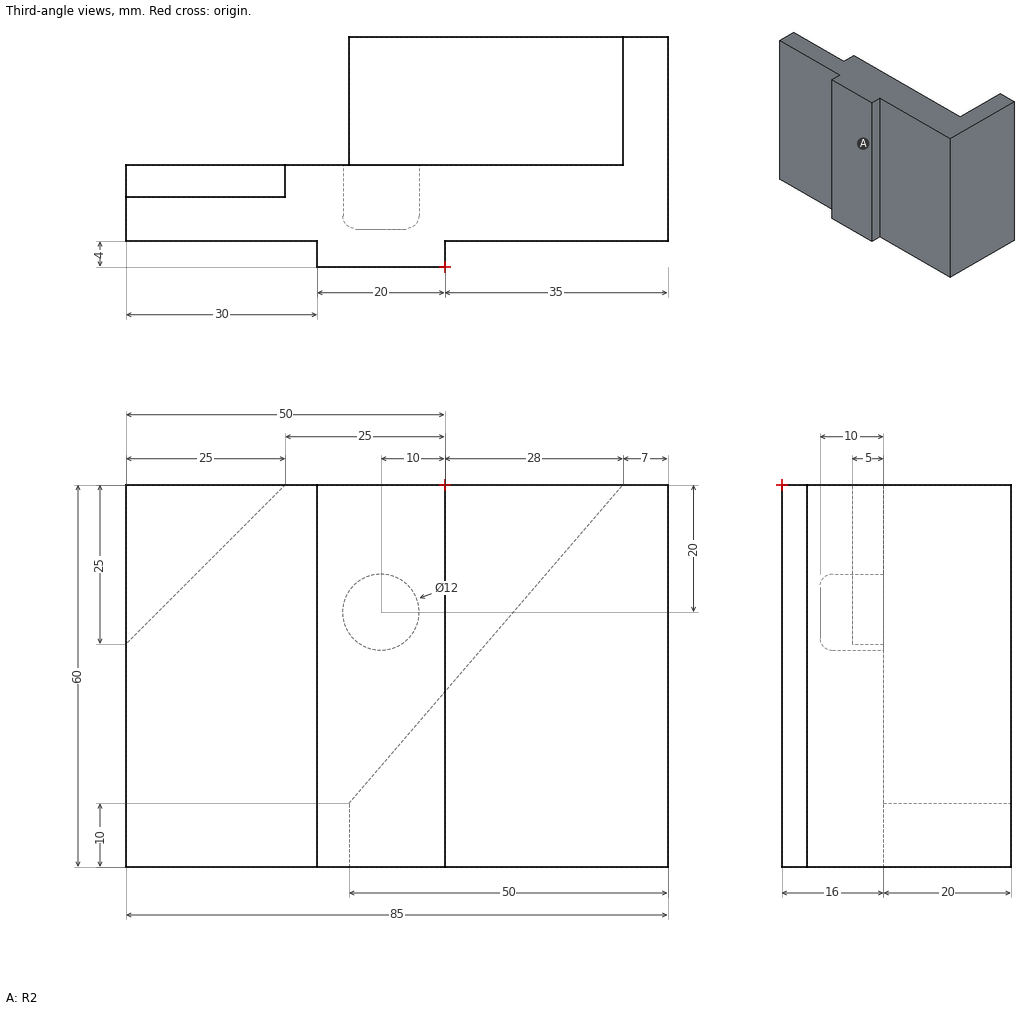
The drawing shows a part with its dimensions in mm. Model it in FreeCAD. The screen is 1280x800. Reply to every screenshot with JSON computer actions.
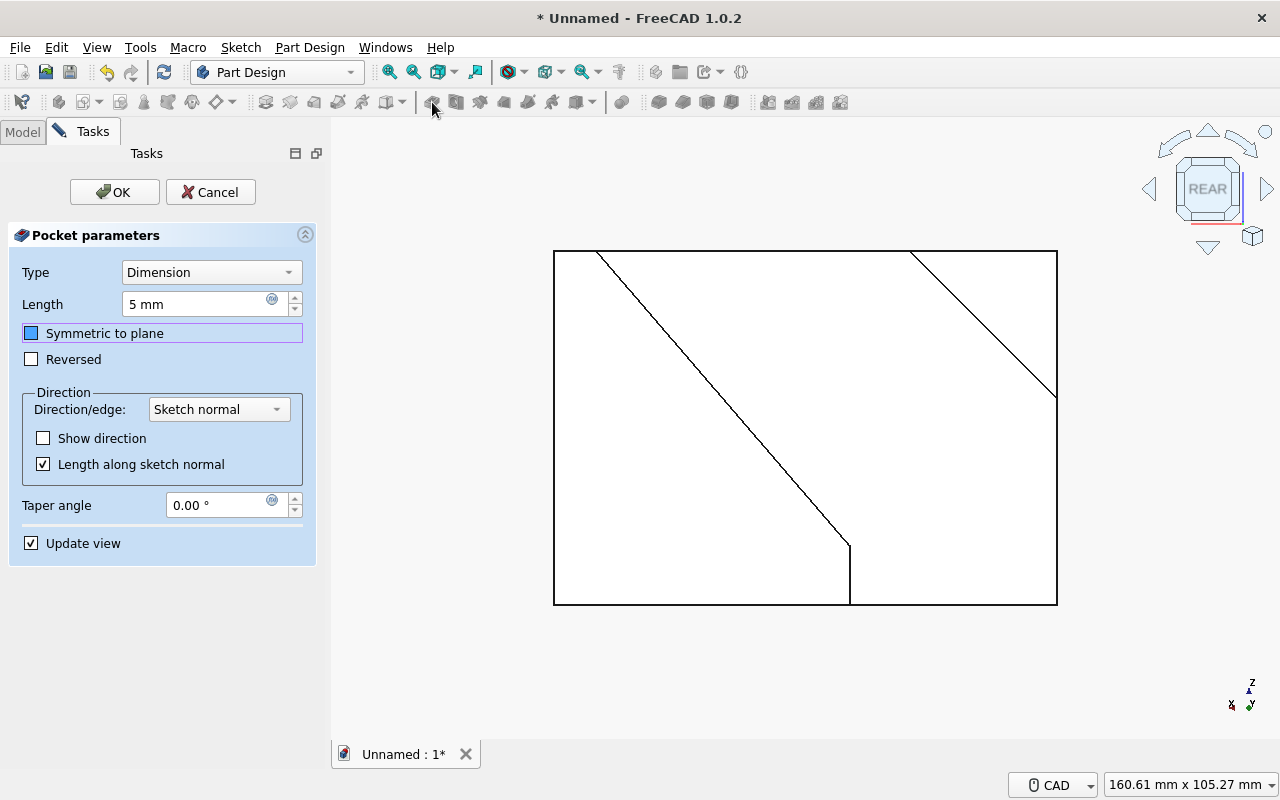
{"action": "left_click", "coordinate": [115, 192]}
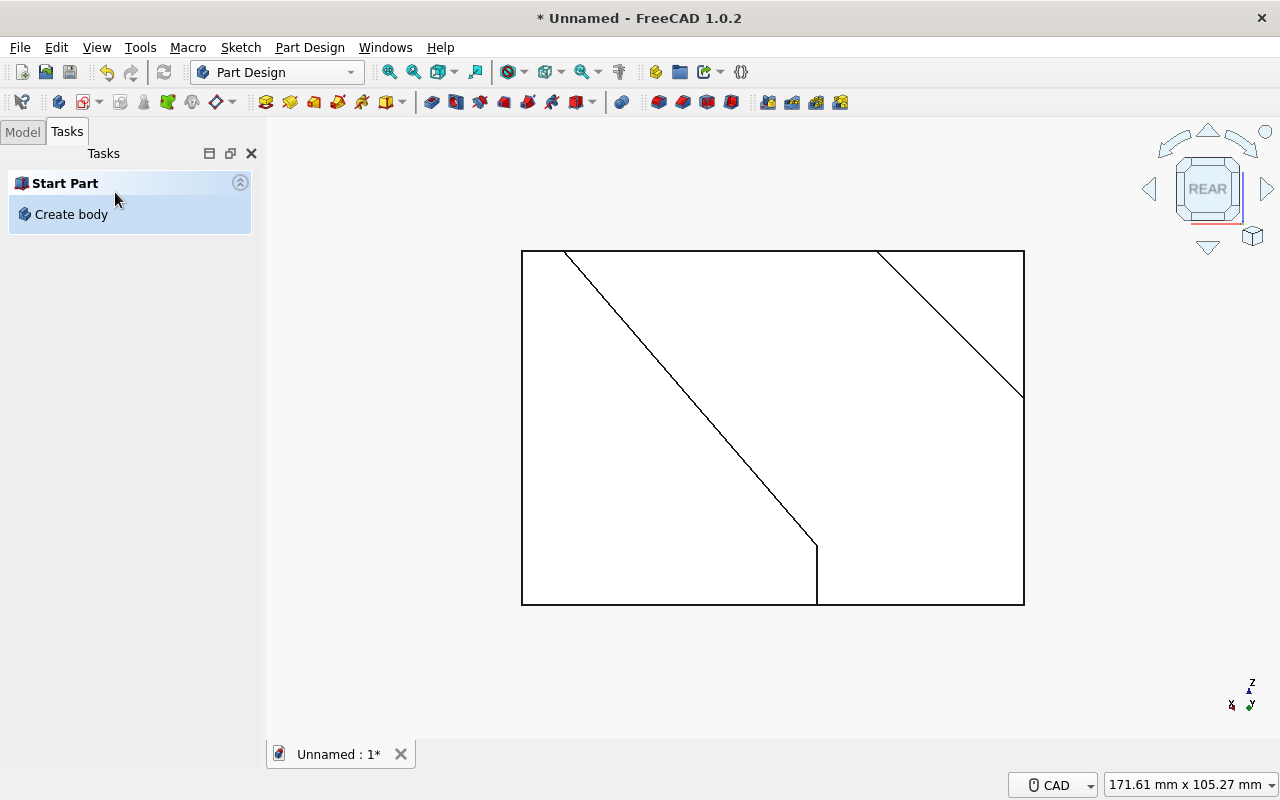
{"action": "left_click", "coordinate": [860, 427]}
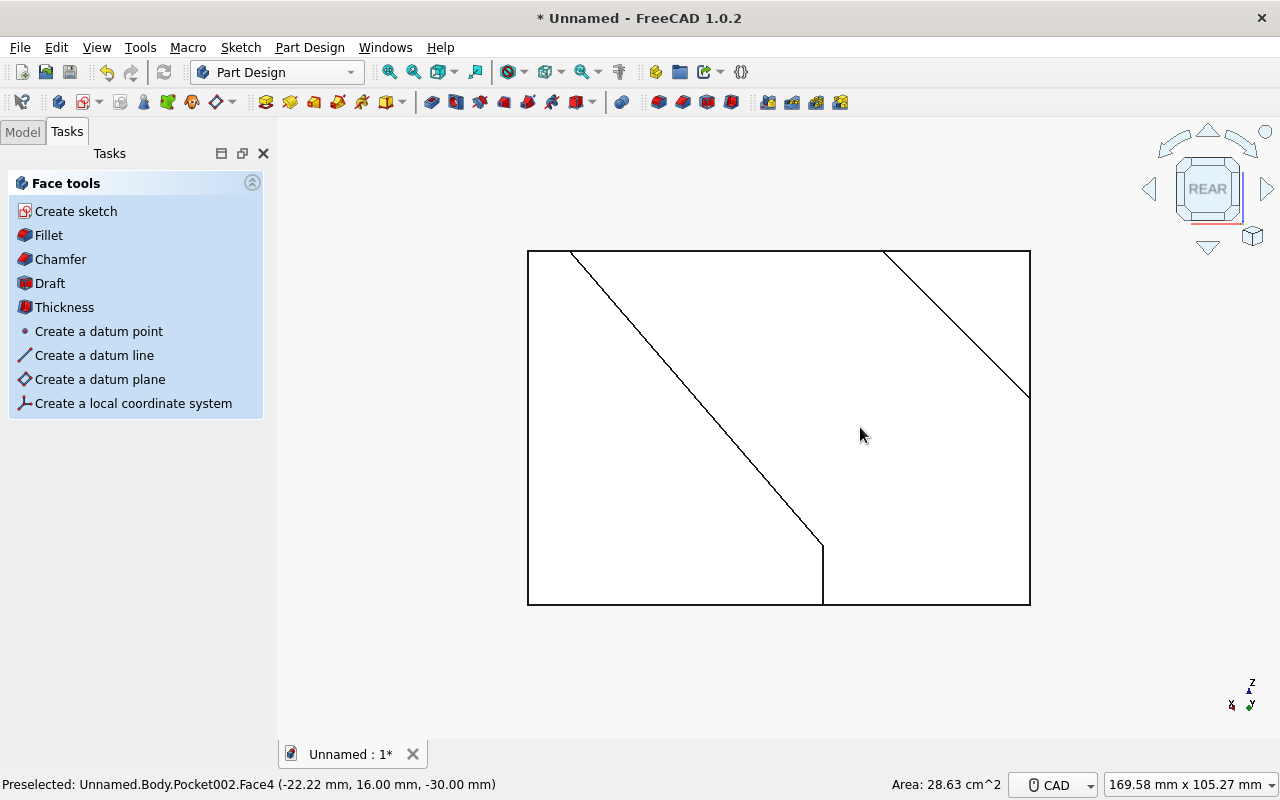
{"action": "left_click", "coordinate": [84, 102]}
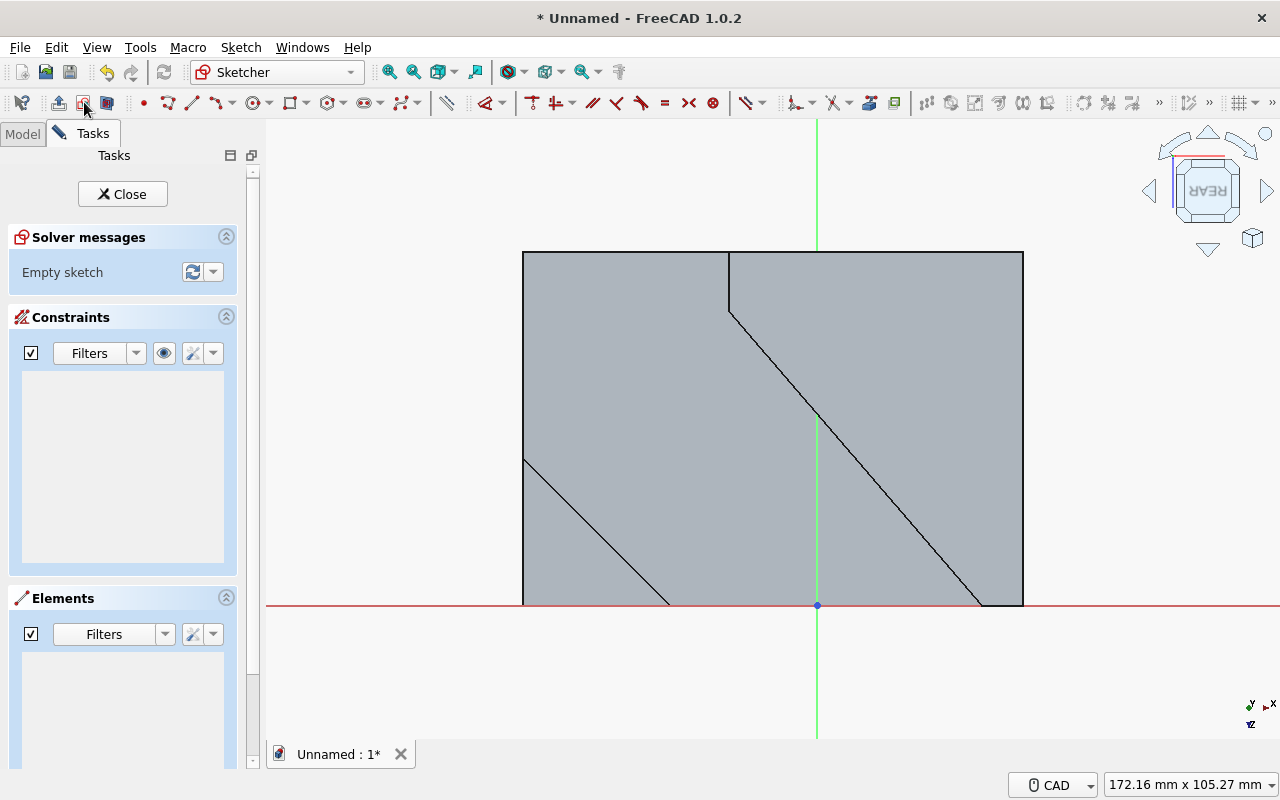
{"action": "scroll", "coordinate": [808, 587], "scroll_direction": "up", "scroll_amount": 5}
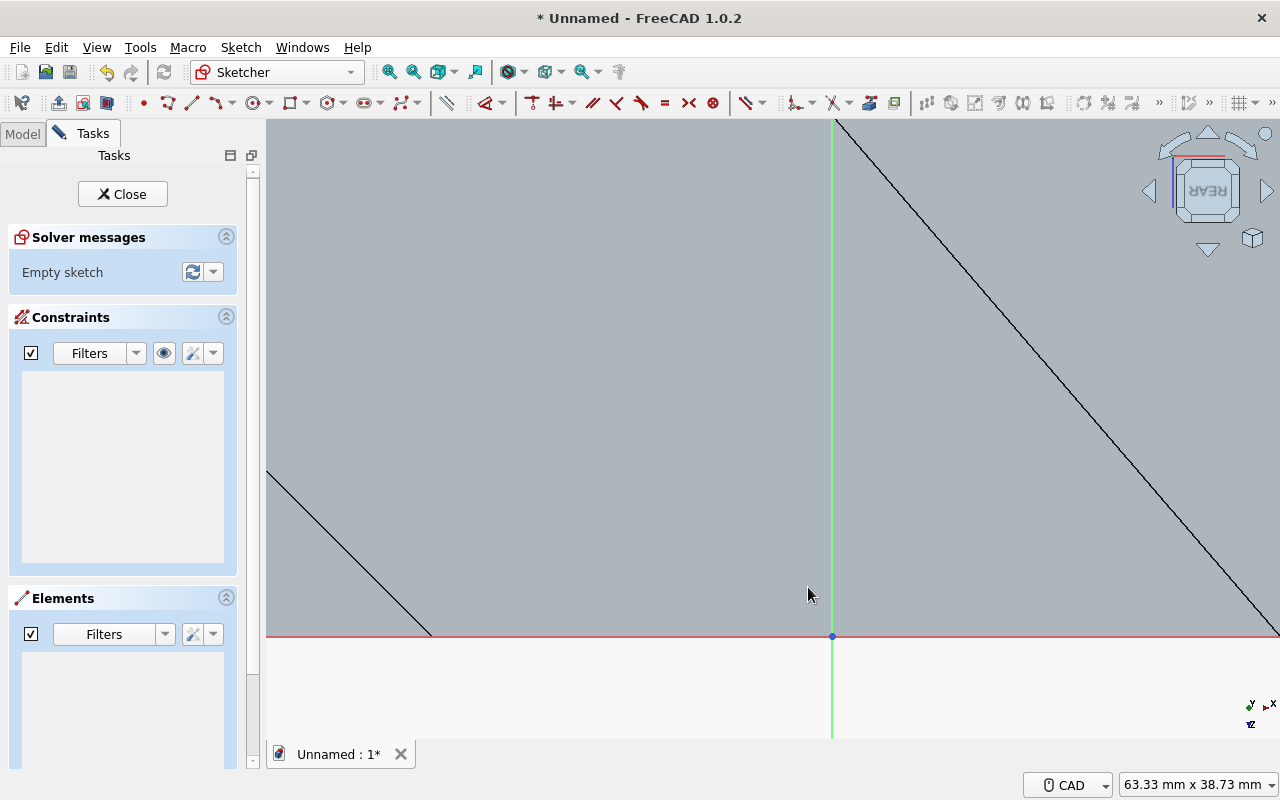
{"action": "left_click", "coordinate": [254, 104]}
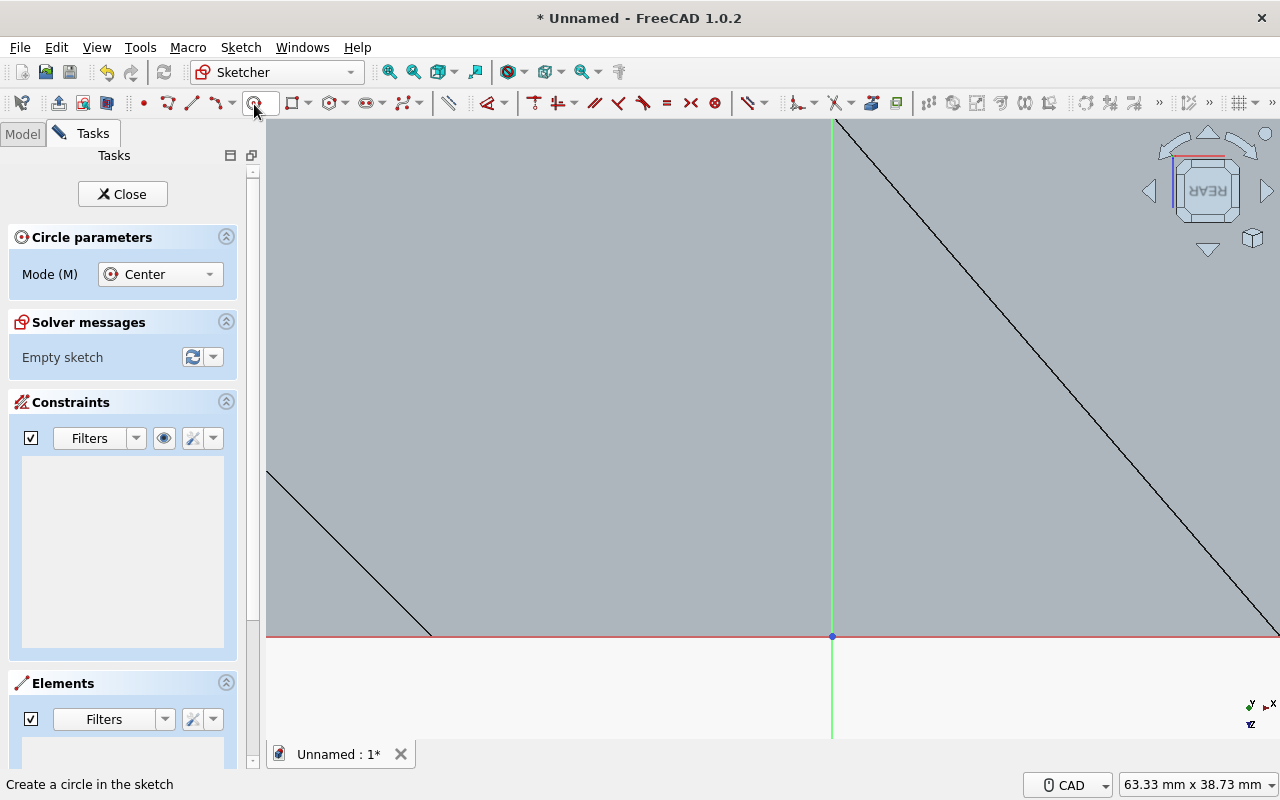
{"action": "left_click", "coordinate": [672, 316]}
{"action": "left_click", "coordinate": [740, 248]}
{"action": "key", "text": "Escape"}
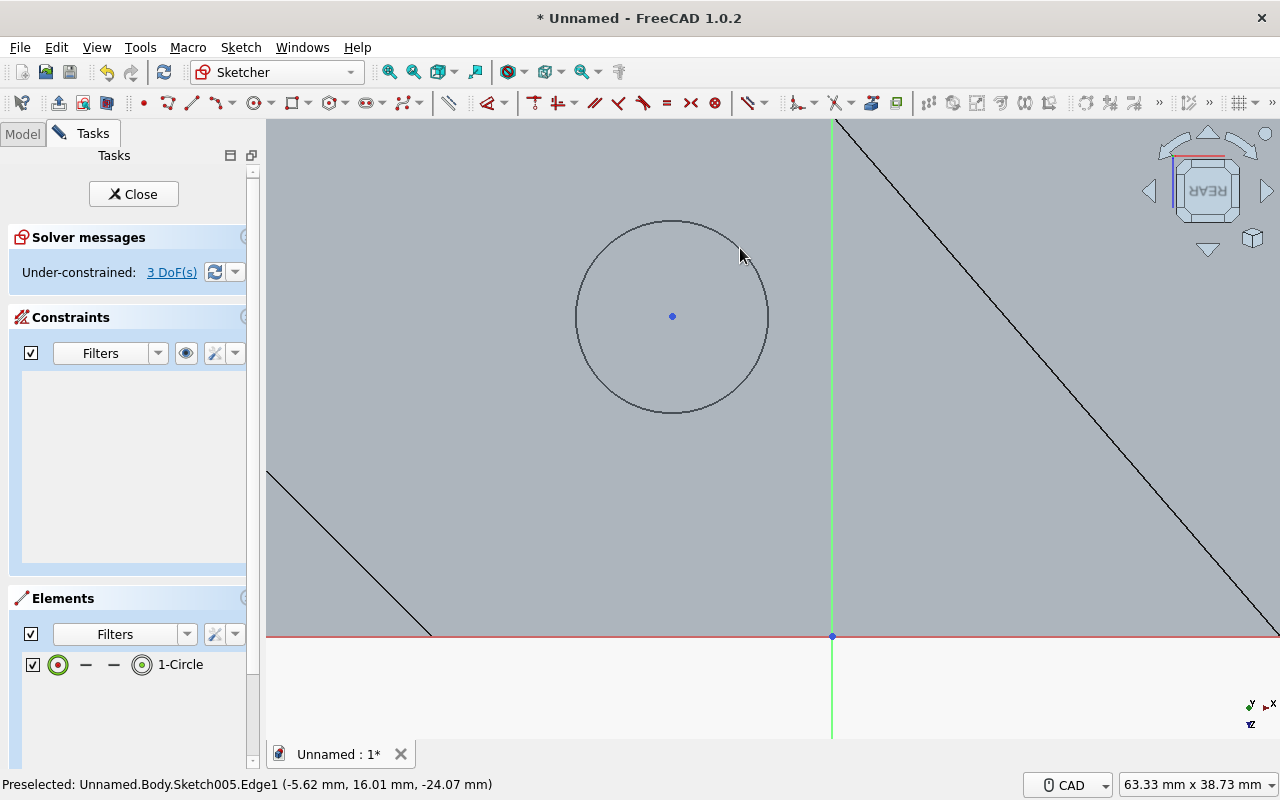
{"action": "left_click", "coordinate": [488, 104]}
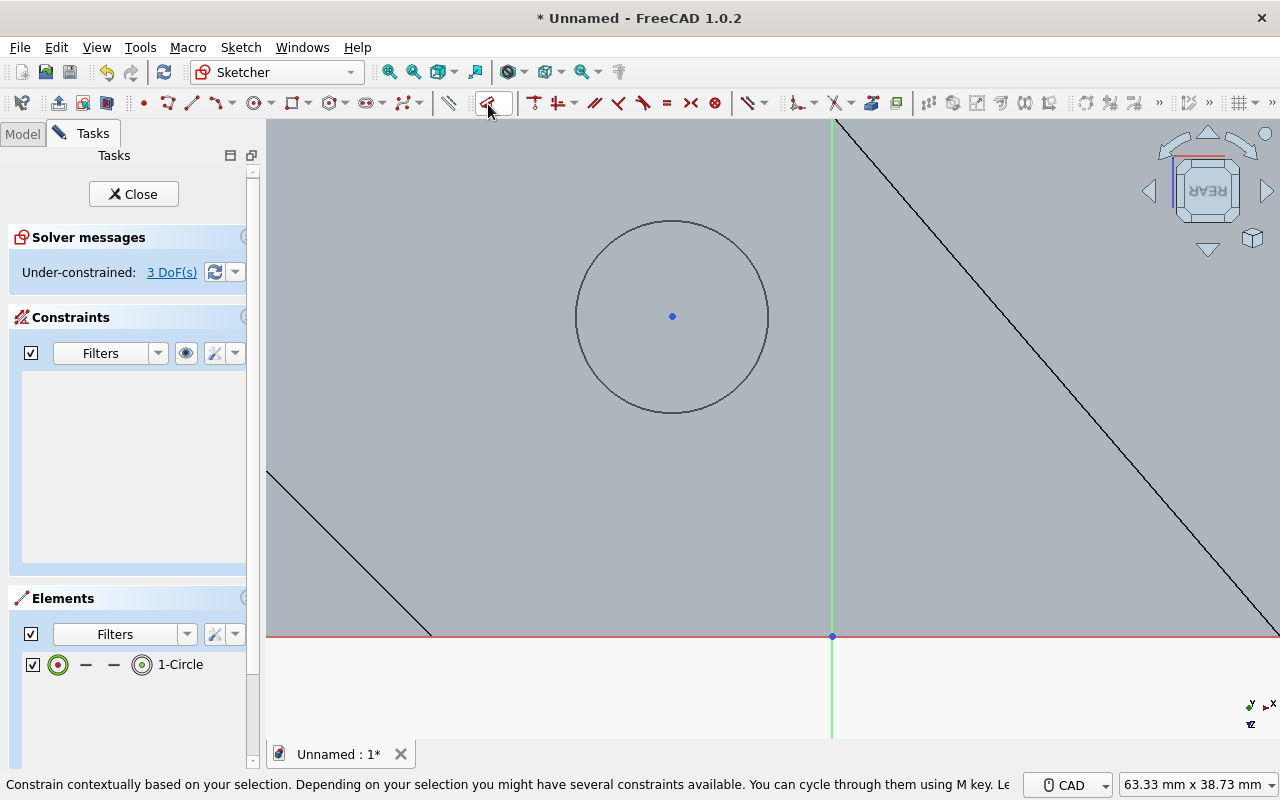
{"action": "left_click", "coordinate": [740, 249]}
{"action": "left_click", "coordinate": [763, 226]}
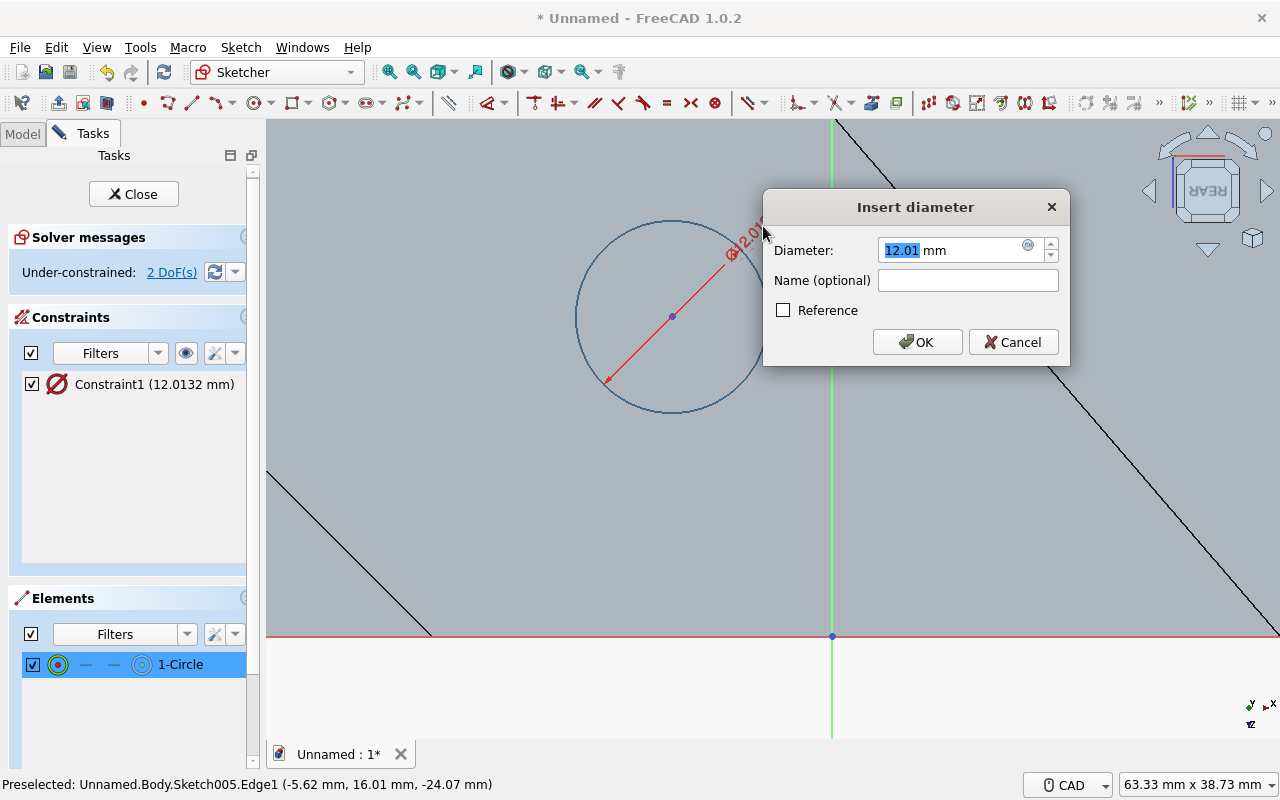
{"action": "type", "text": "12"}
{"action": "key", "text": "Return"}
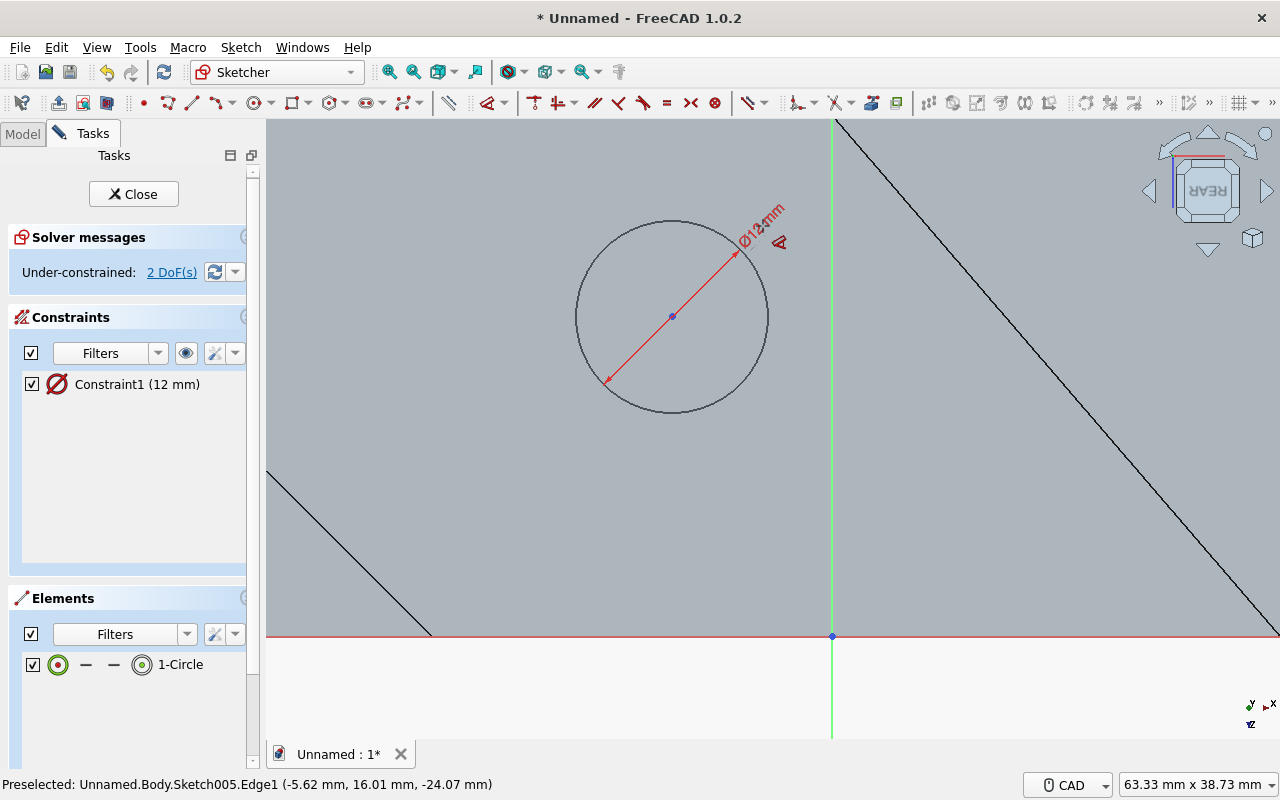
{"action": "left_click", "coordinate": [672, 317]}
{"action": "left_click", "coordinate": [752, 671]}